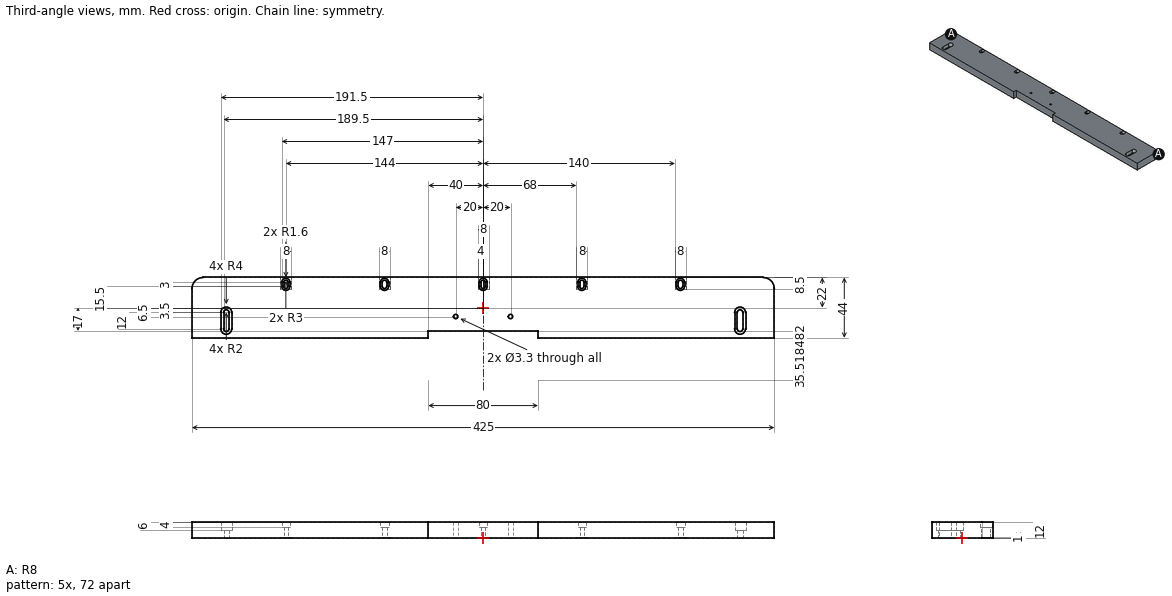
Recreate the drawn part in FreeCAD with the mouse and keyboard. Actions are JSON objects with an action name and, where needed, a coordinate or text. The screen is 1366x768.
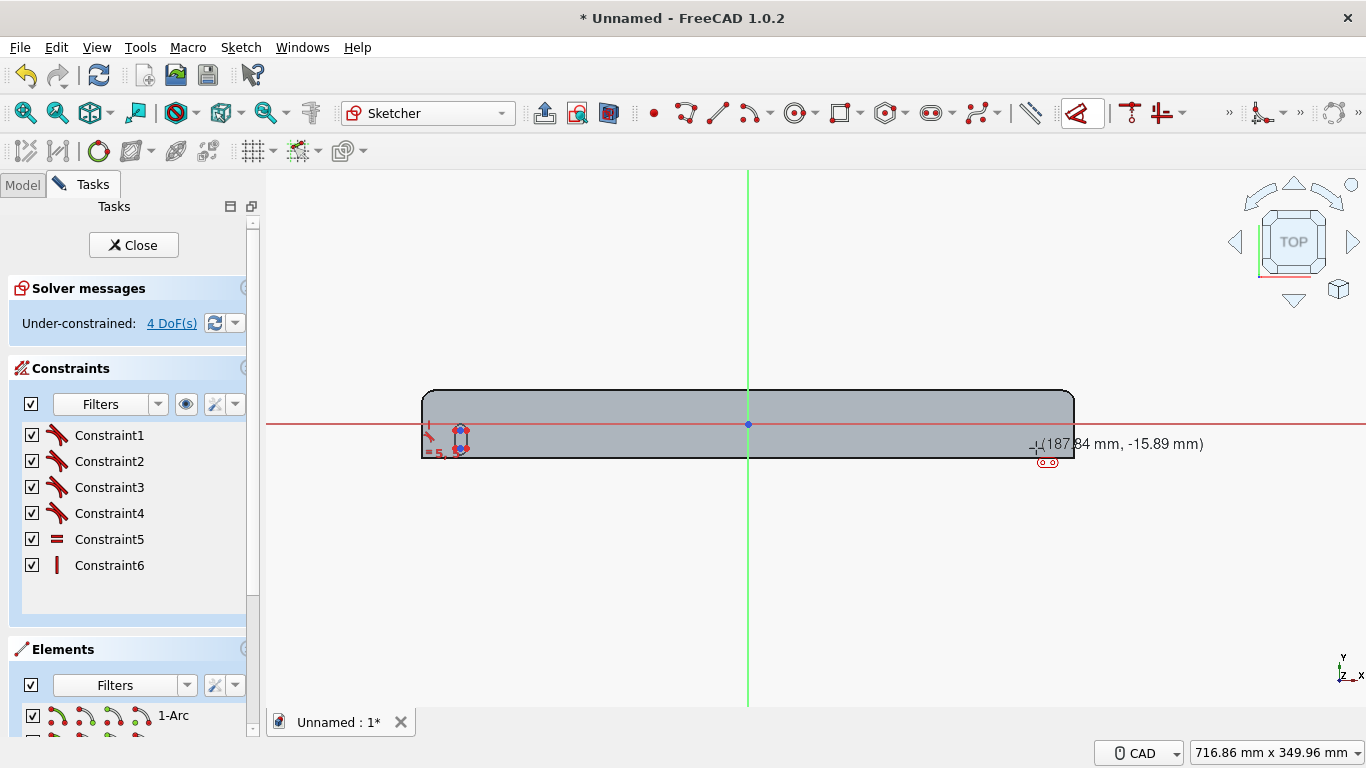
{"action": "left_click", "coordinate": [1036, 448]}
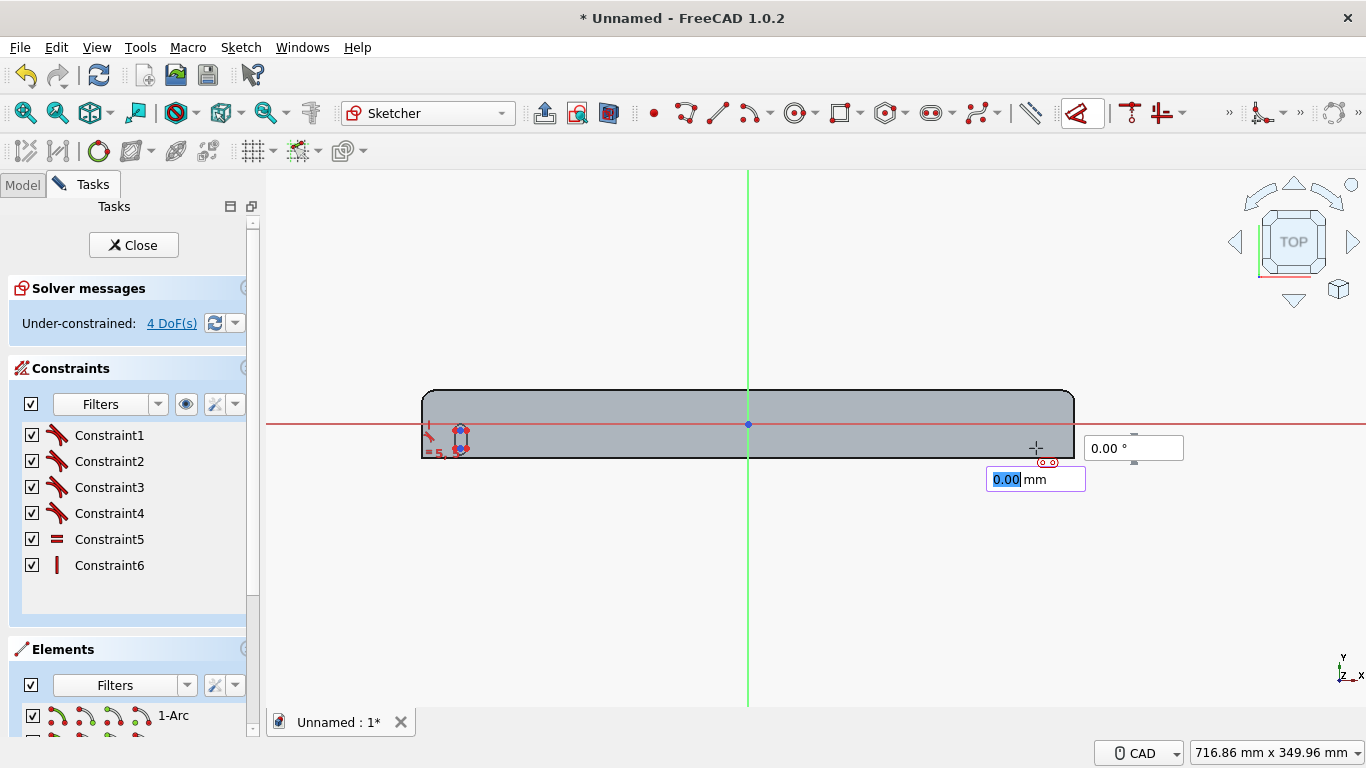
{"action": "scroll", "coordinate": [1036, 430], "scroll_direction": "up", "scroll_amount": 6}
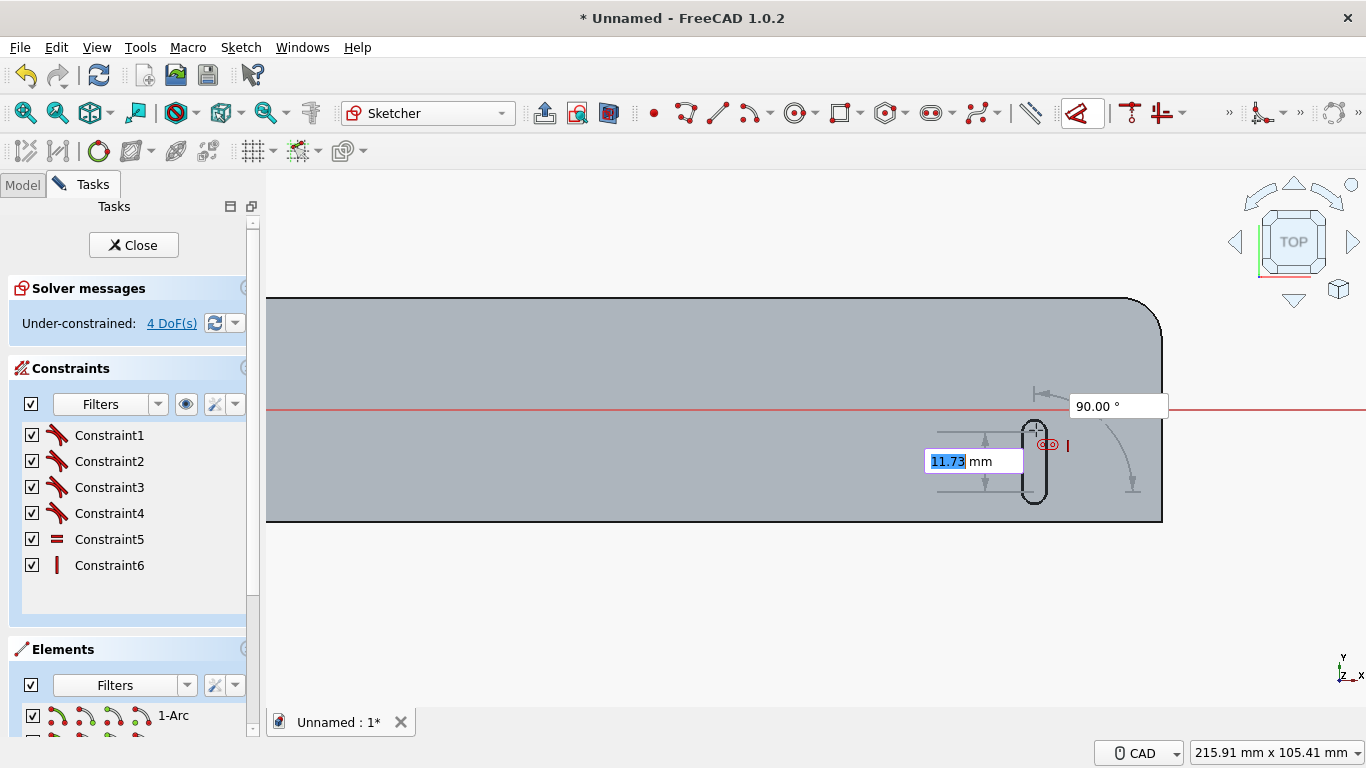
{"action": "left_click", "coordinate": [1034, 428]}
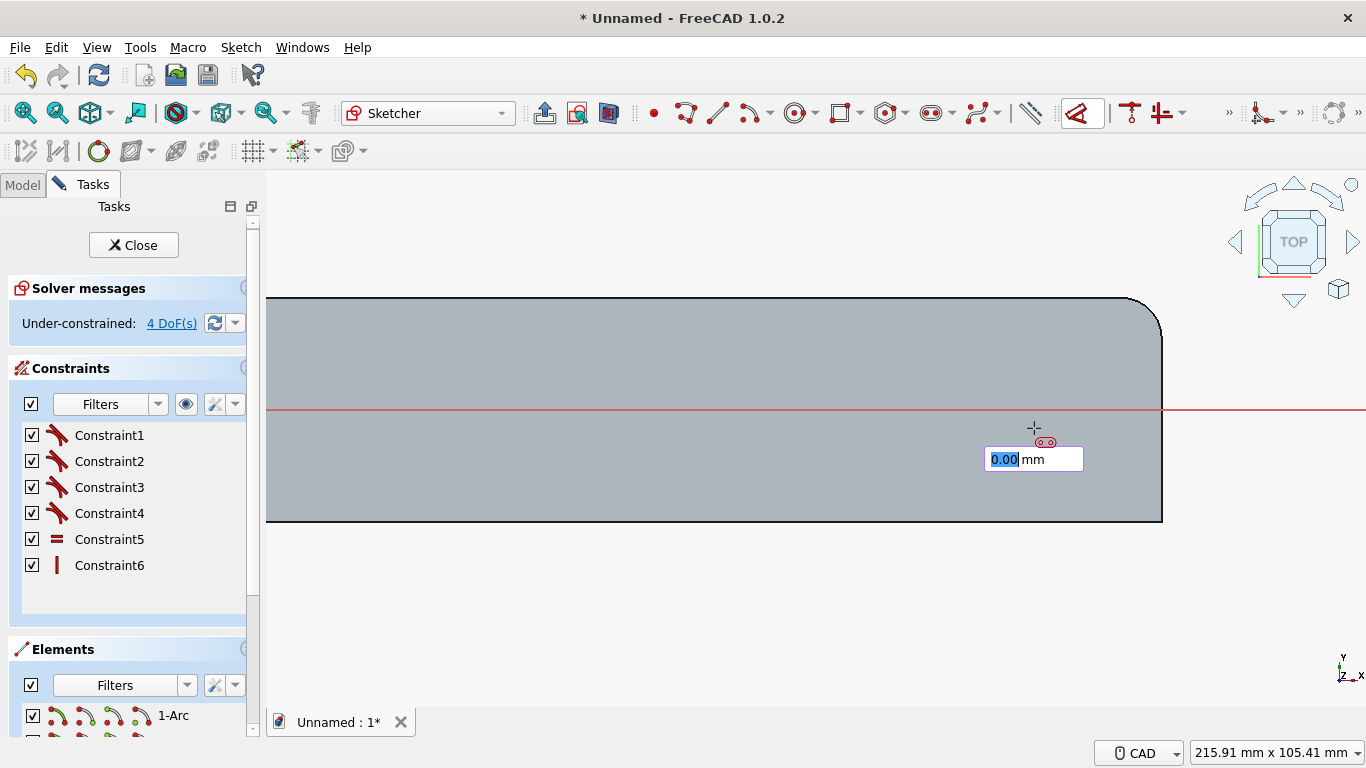
{"action": "left_click", "coordinate": [1014, 458]}
{"action": "key", "text": "Escape"}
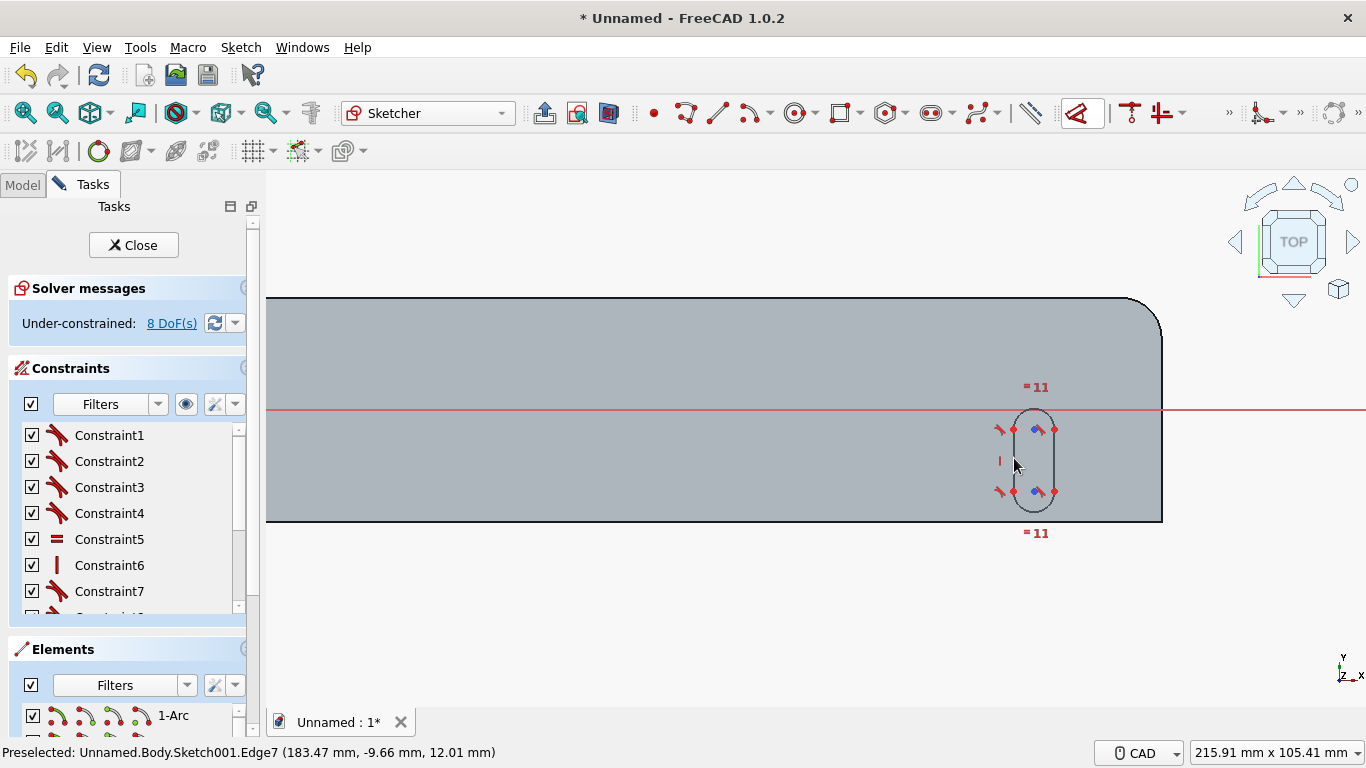
{"action": "scroll", "coordinate": [1036, 430], "scroll_direction": "down", "scroll_amount": 6}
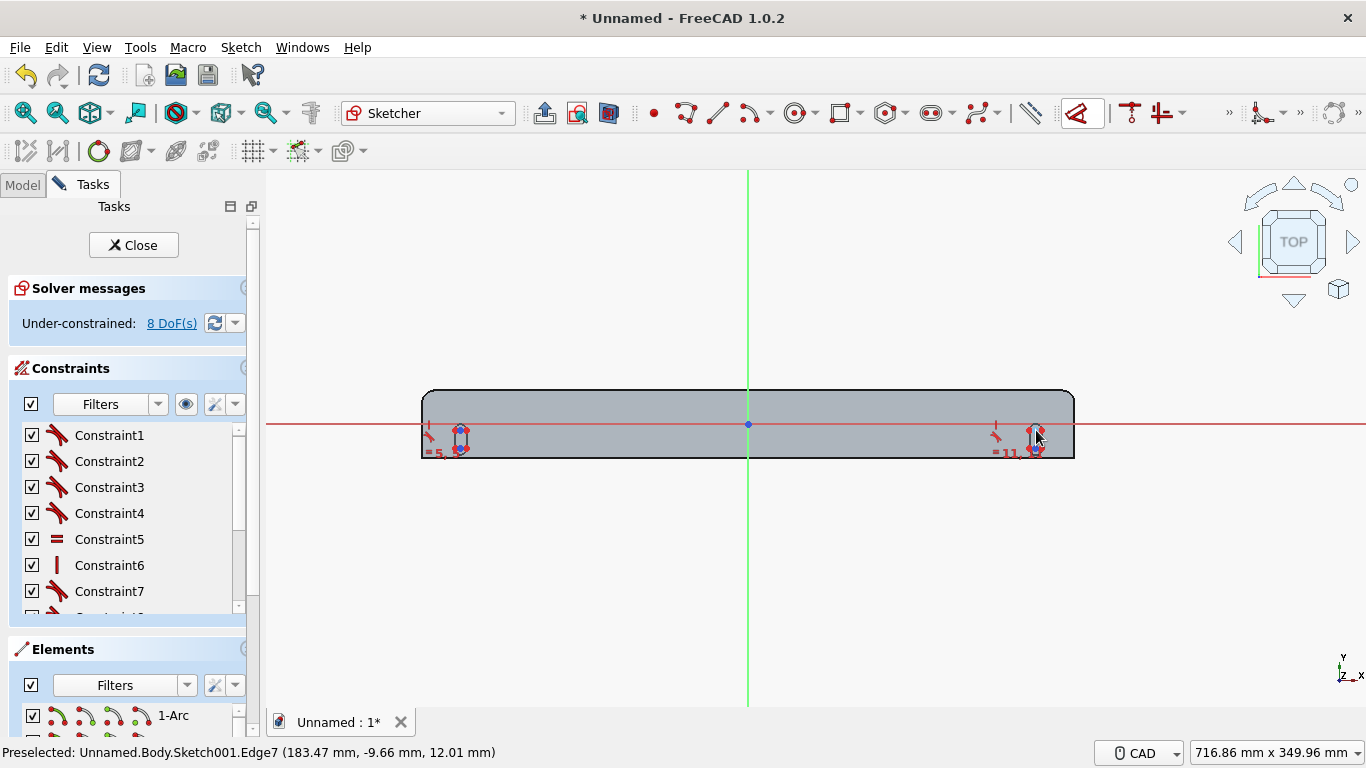
{"action": "scroll", "coordinate": [457, 454], "scroll_direction": "up", "scroll_amount": 5}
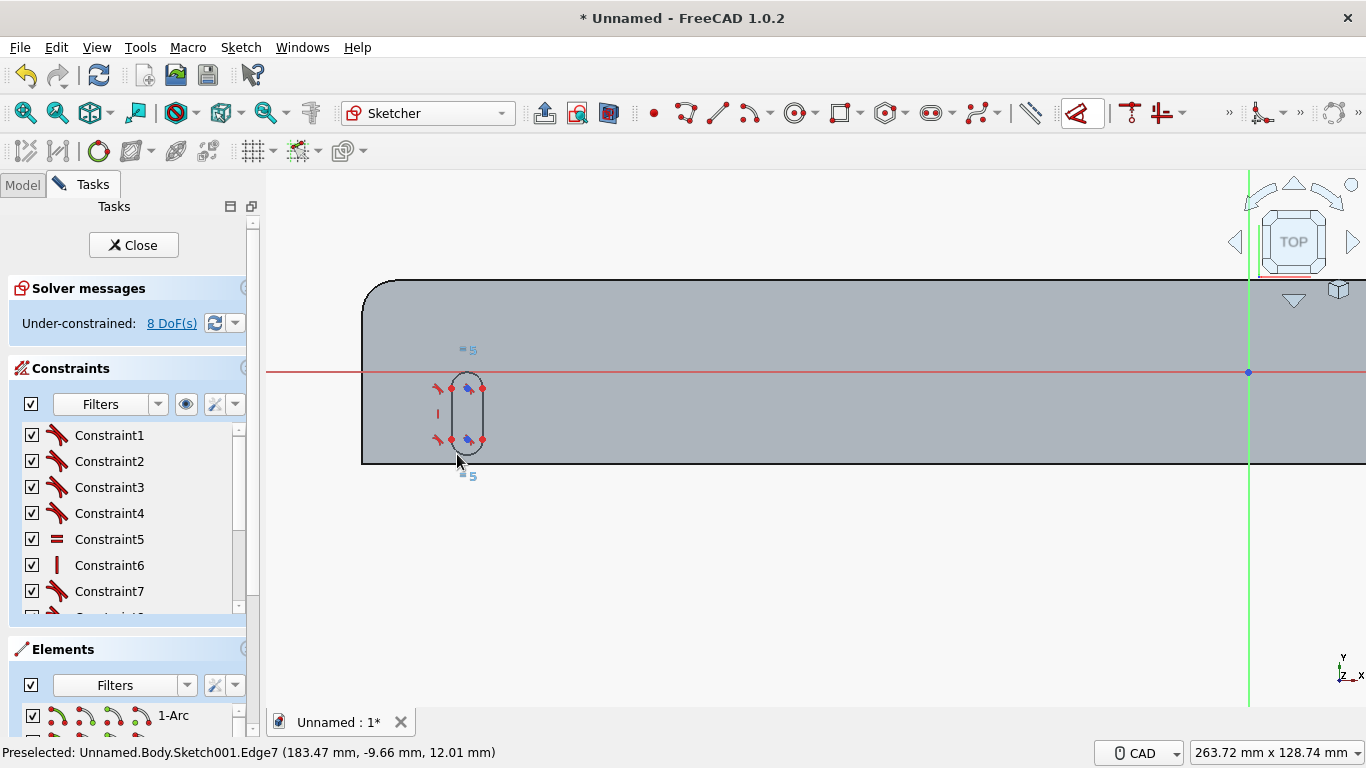
{"action": "left_click", "coordinate": [458, 452]}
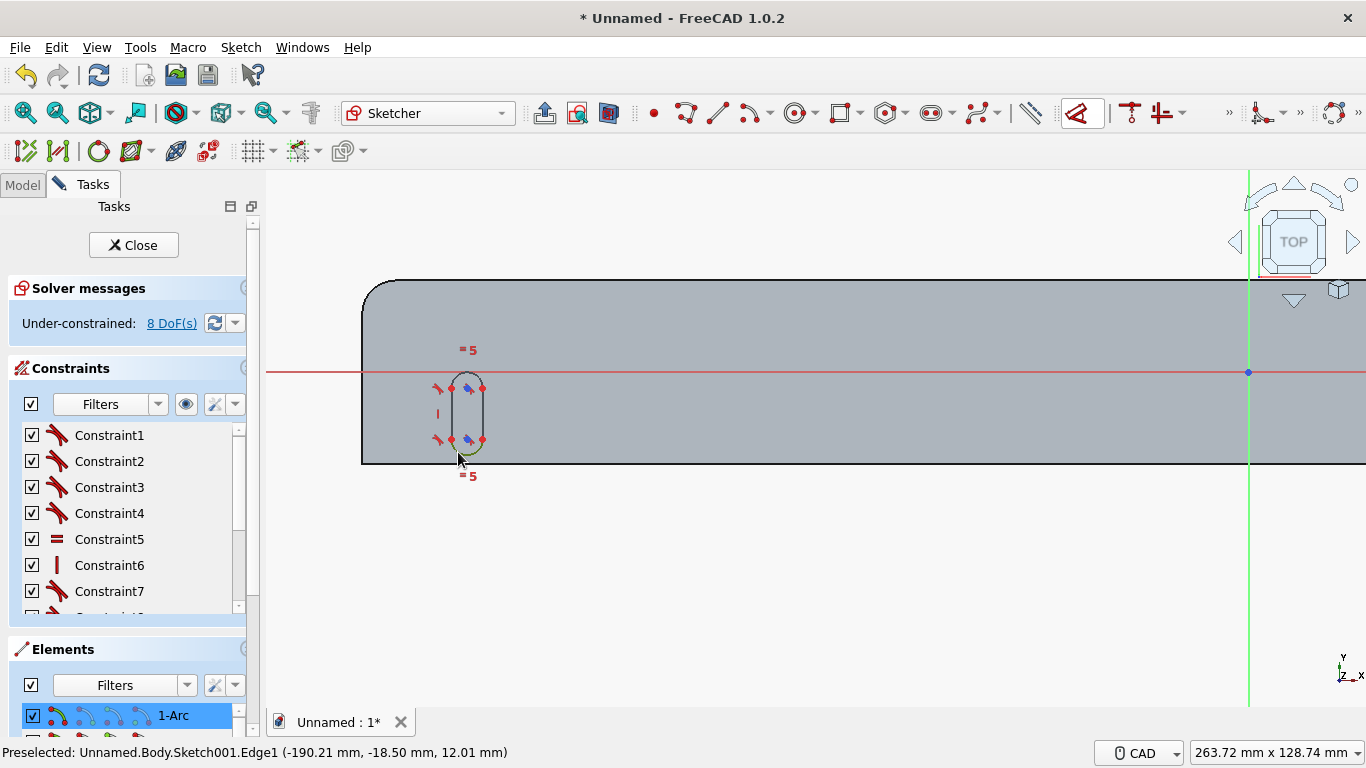
{"action": "scroll", "coordinate": [456, 454], "scroll_direction": "down", "scroll_amount": 5}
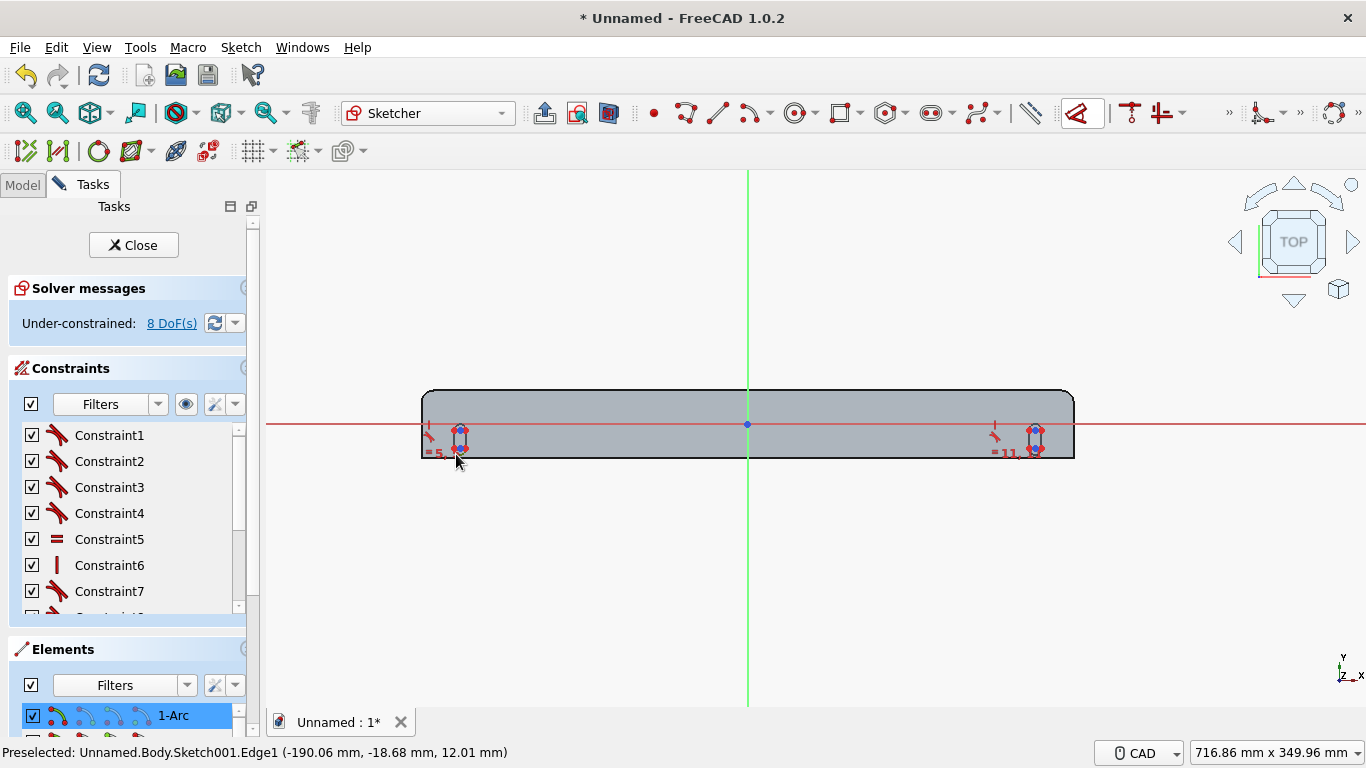
{"action": "scroll", "coordinate": [1032, 454], "scroll_direction": "up", "scroll_amount": 5}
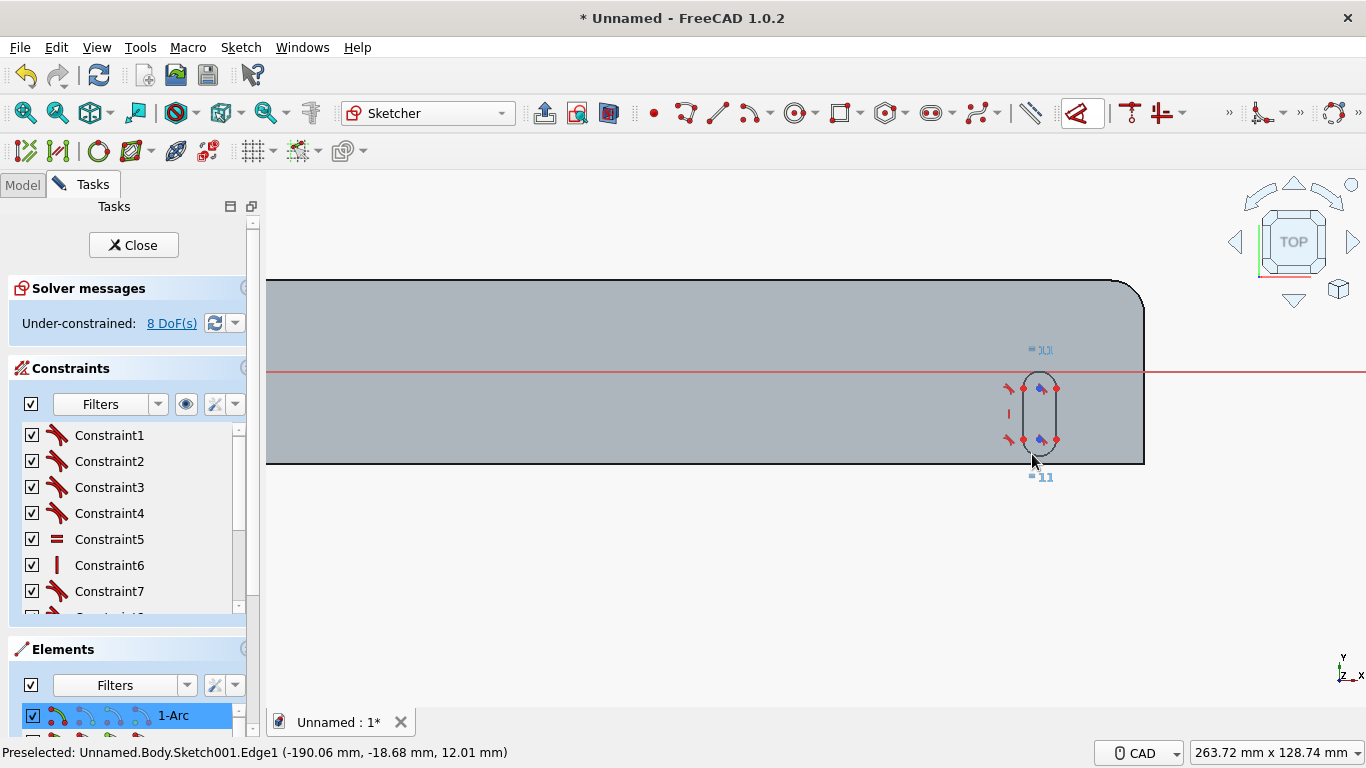
{"action": "left_click", "coordinate": [1030, 453]}